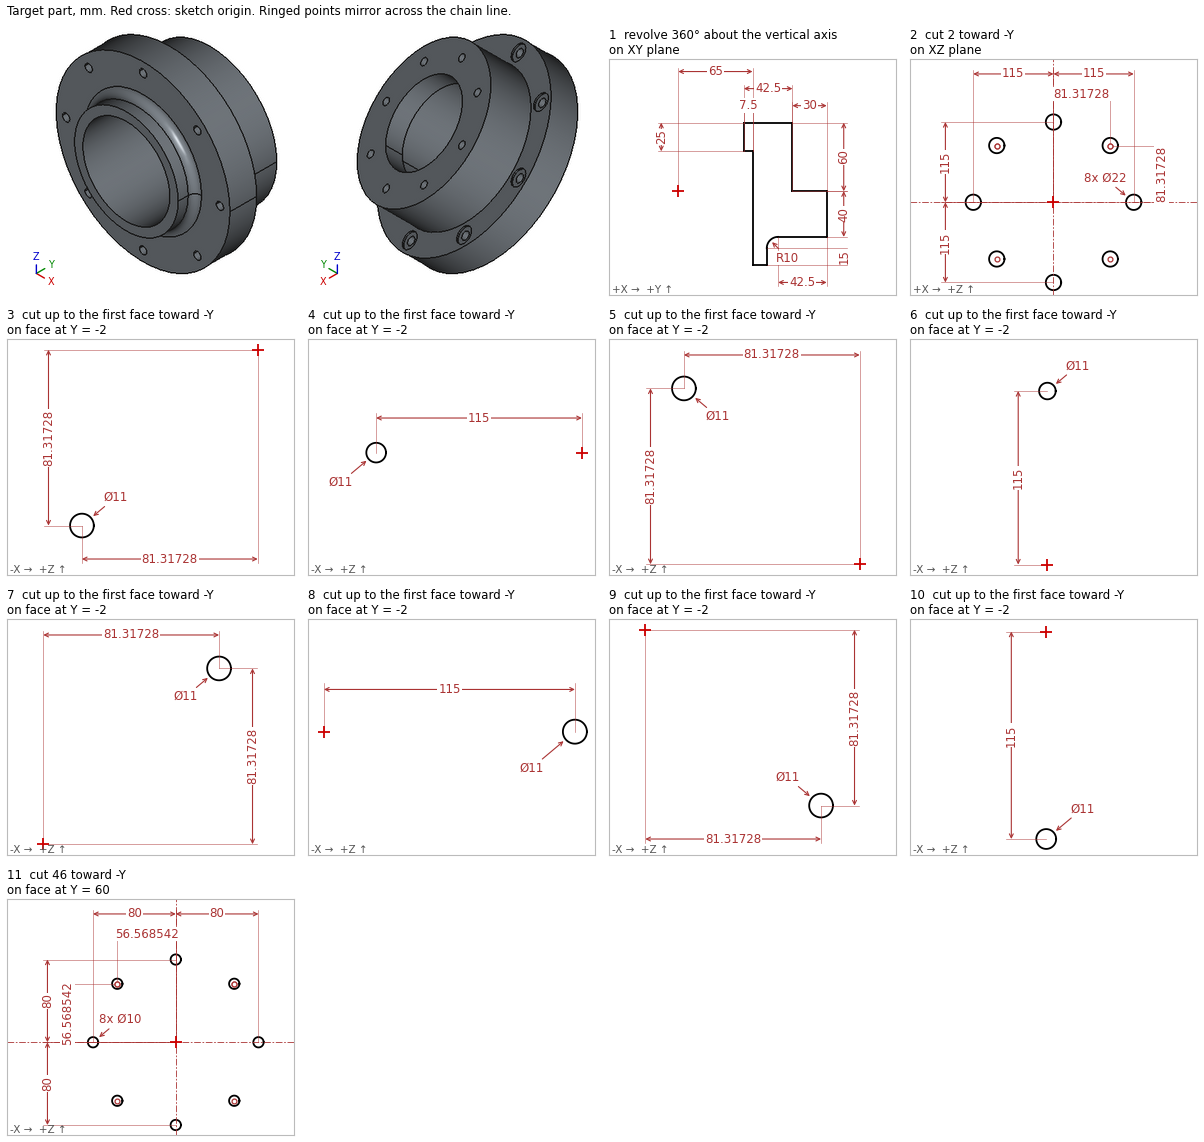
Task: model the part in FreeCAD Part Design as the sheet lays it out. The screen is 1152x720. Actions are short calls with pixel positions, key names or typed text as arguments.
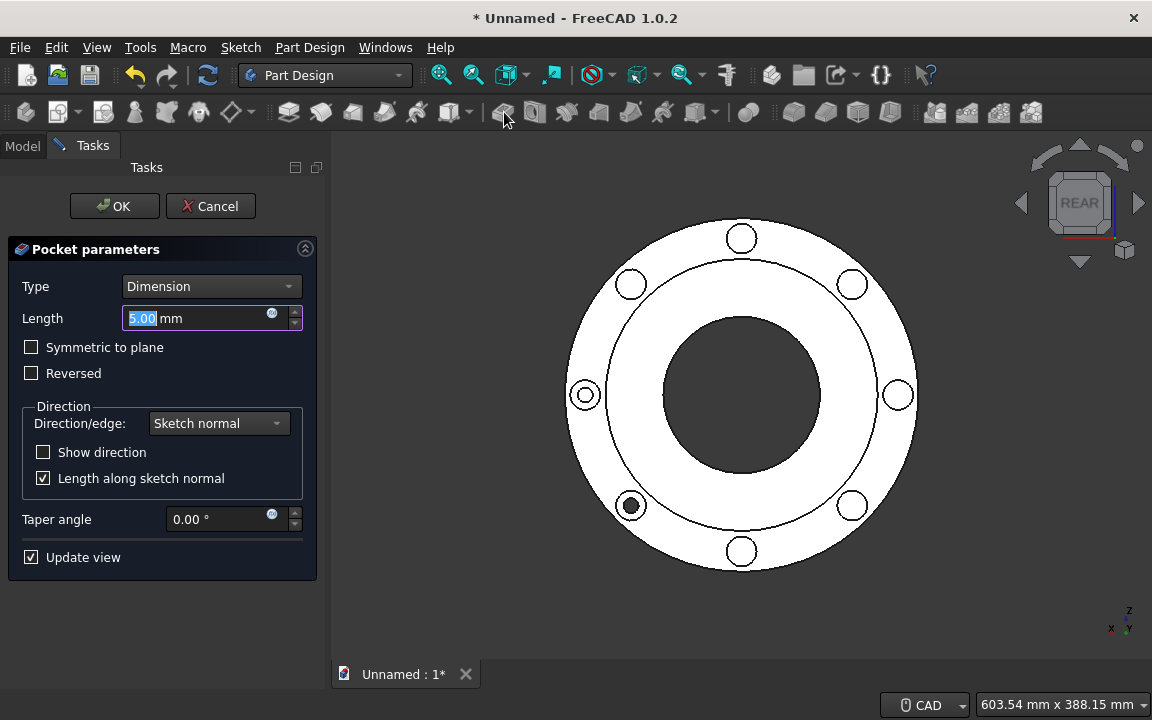
click(212, 286)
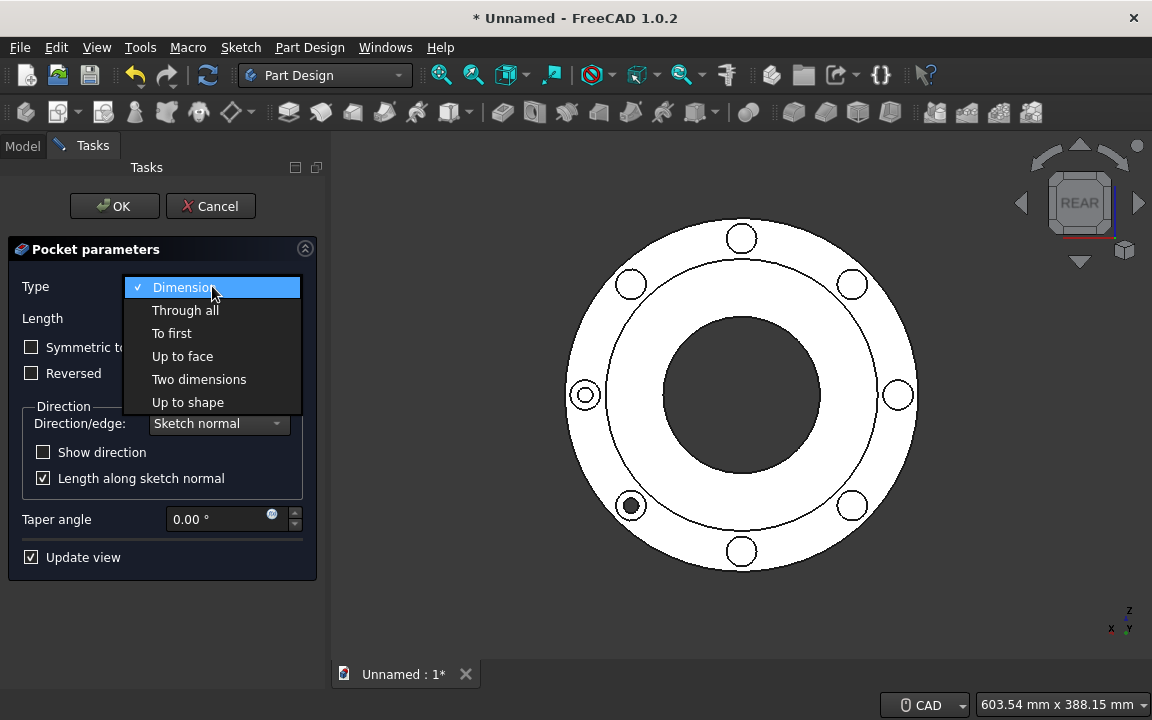
click(212, 334)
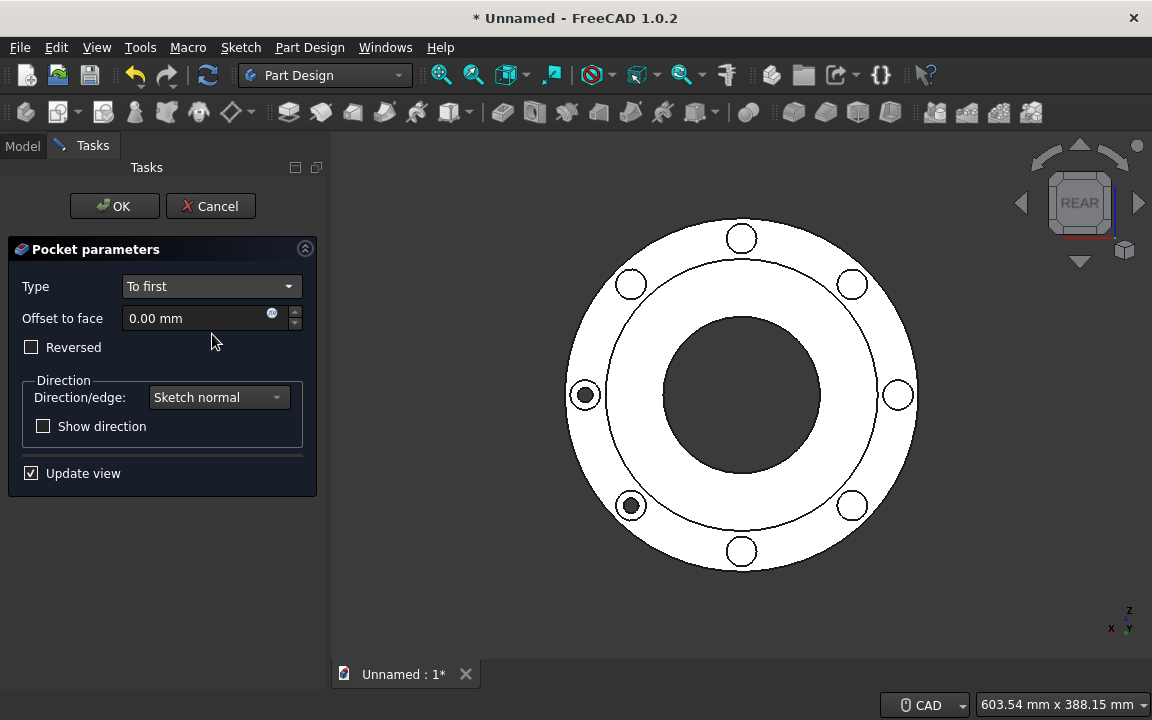
click(115, 206)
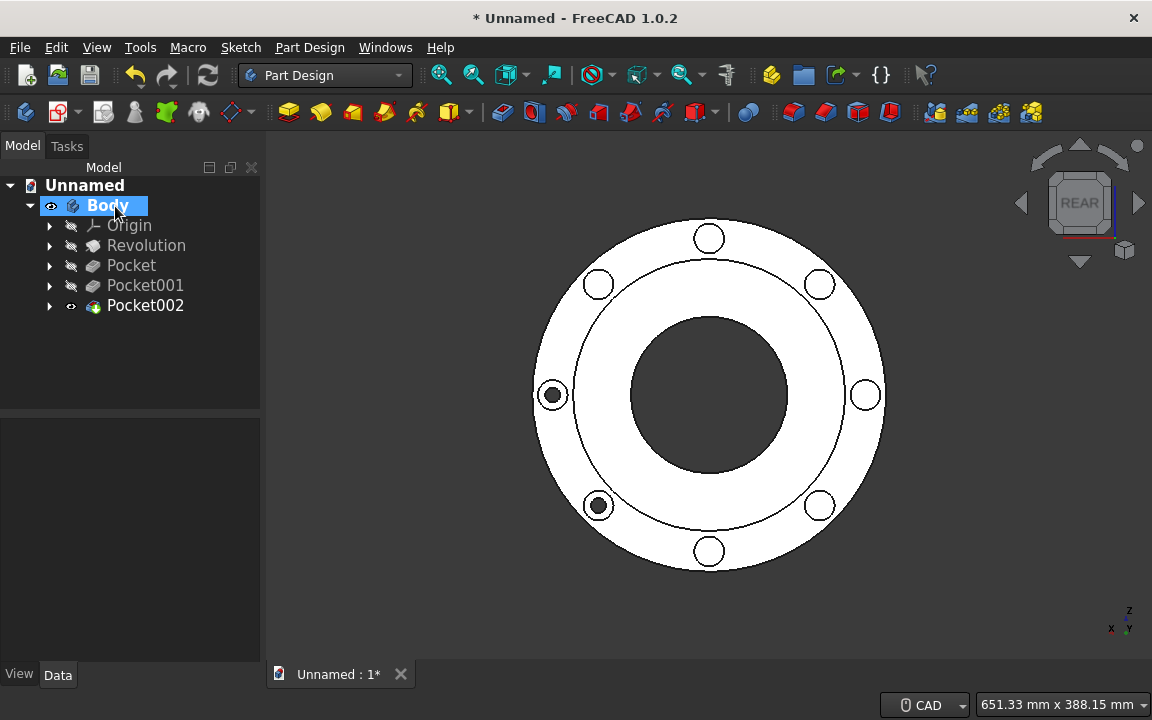
click(599, 283)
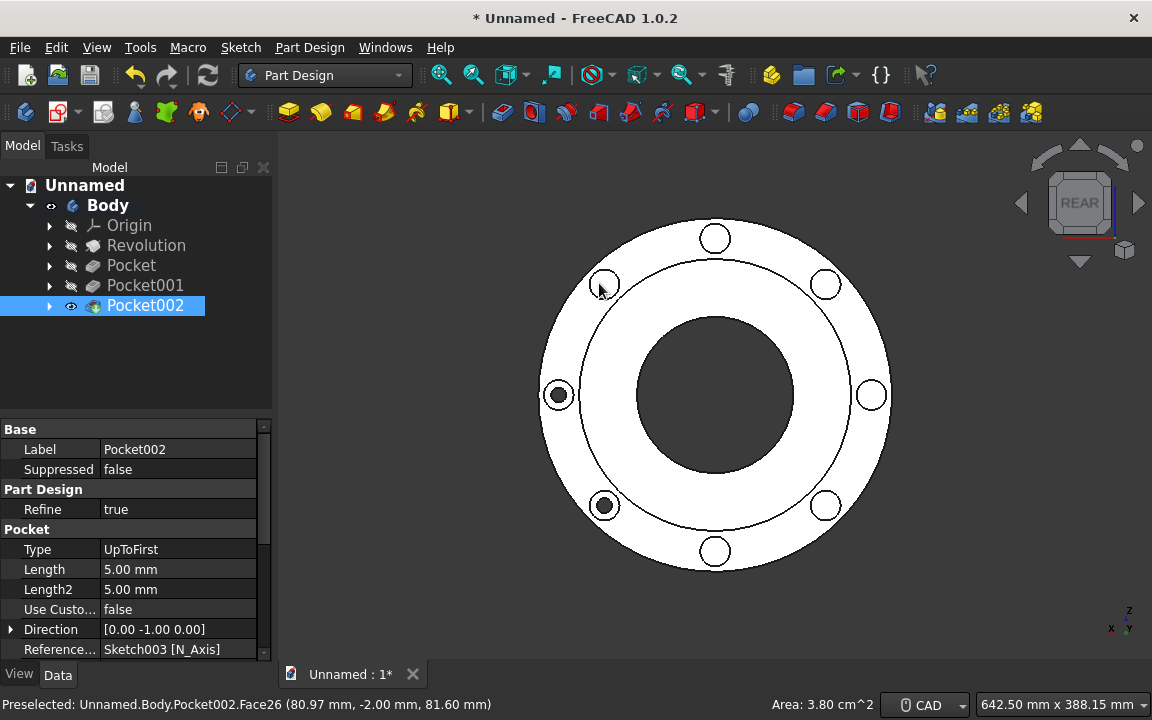
click(58, 112)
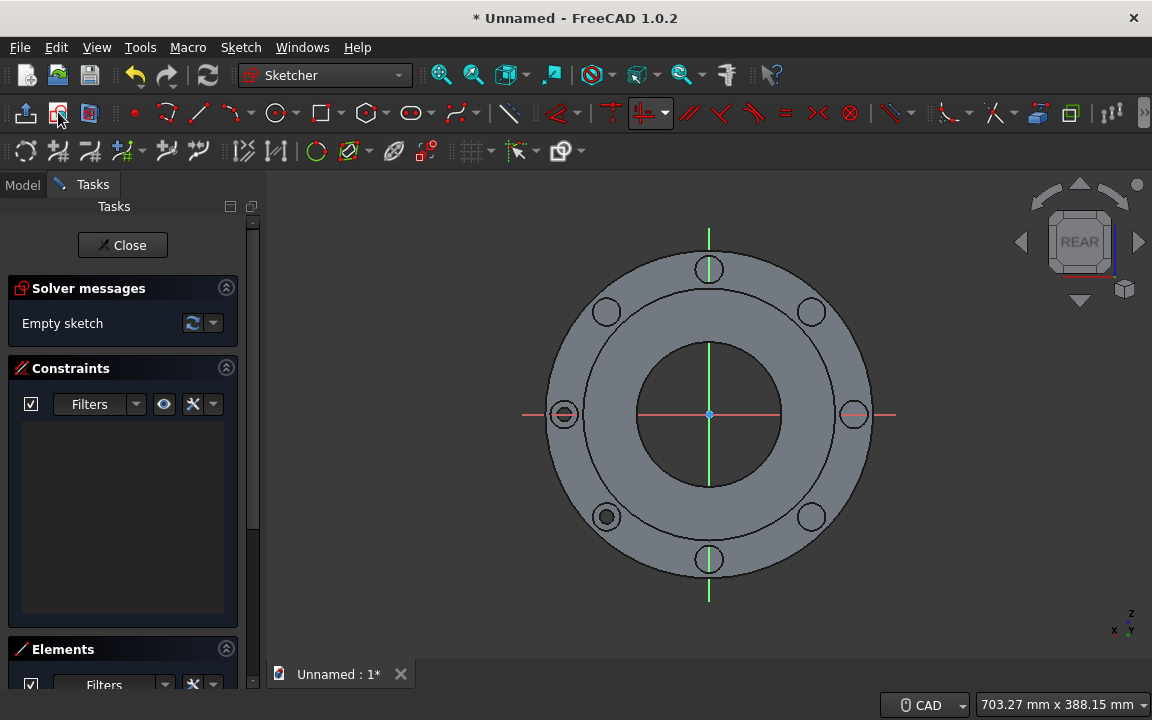
scroll(605, 307, up, 15)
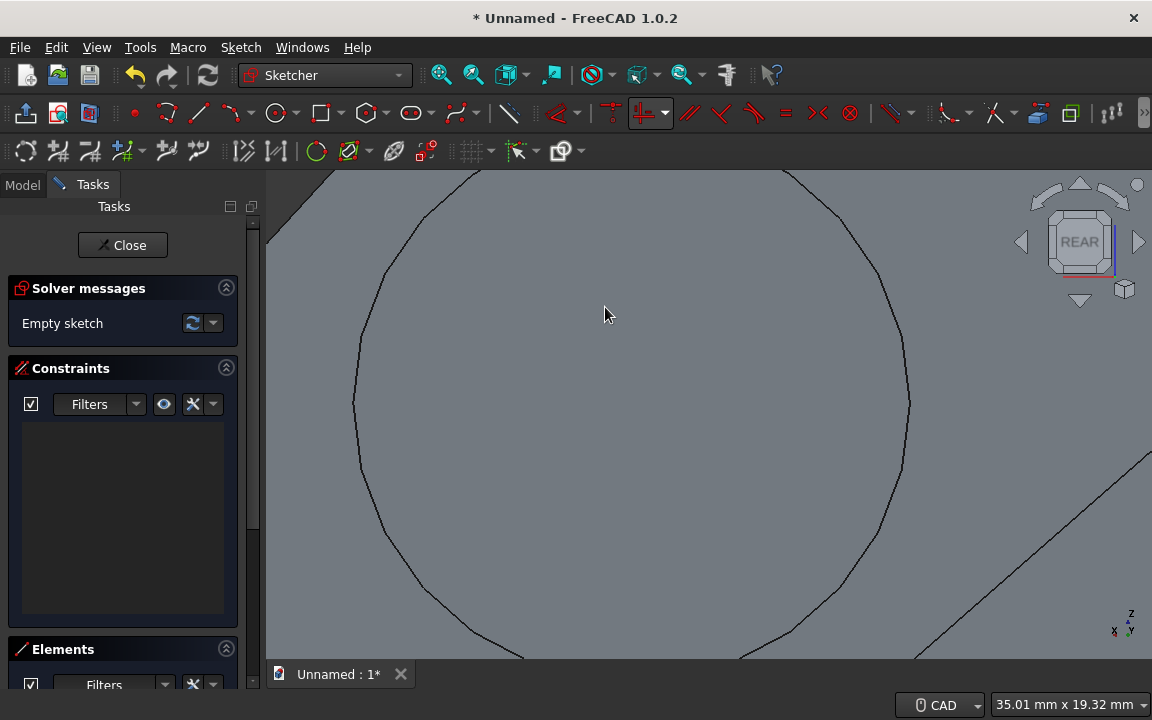
click(276, 114)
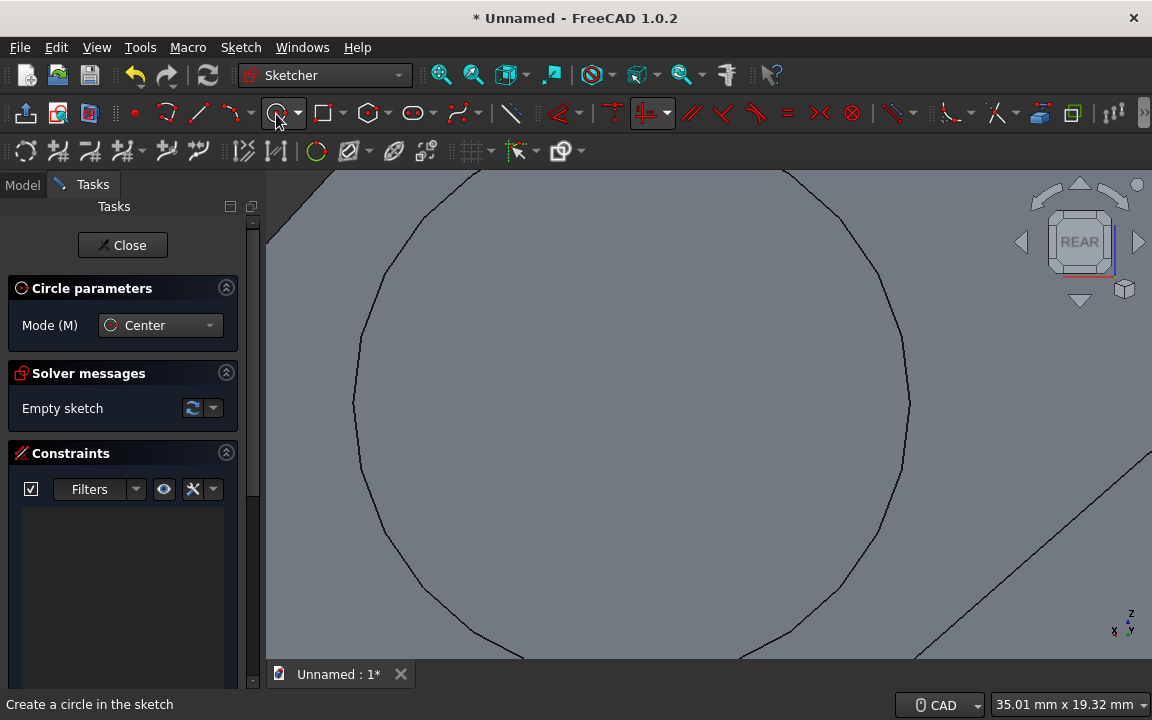
click(632, 403)
move(730, 305)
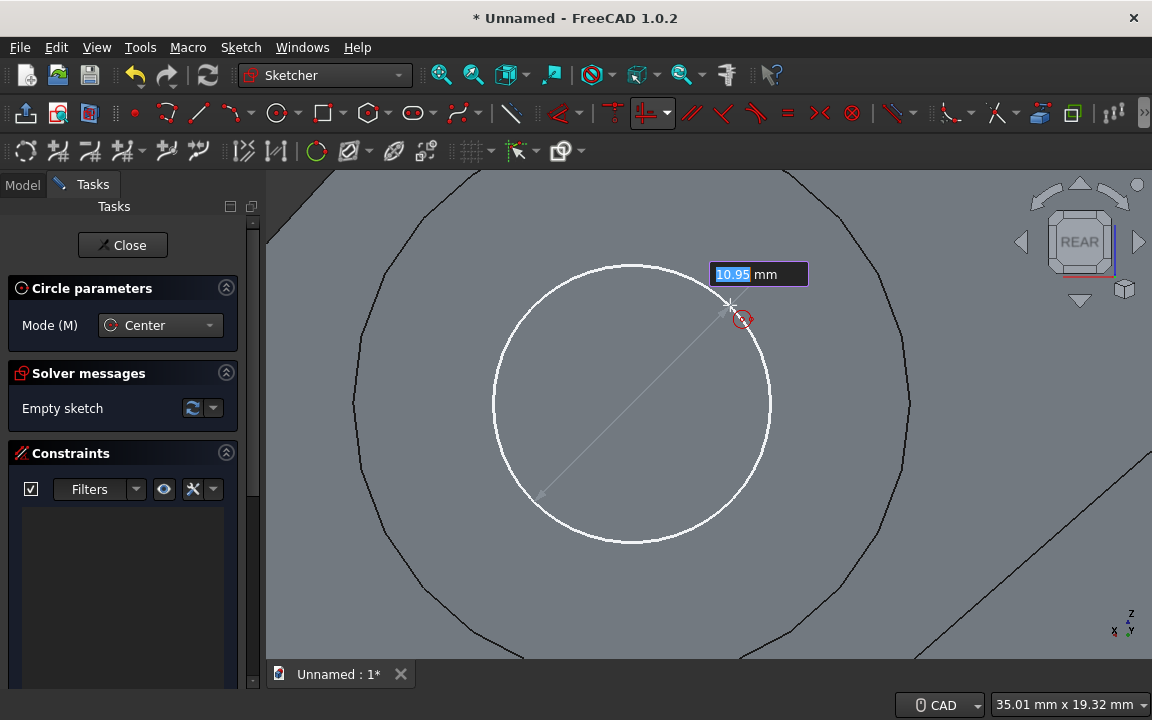
text(11)
key(Return)
key(Escape)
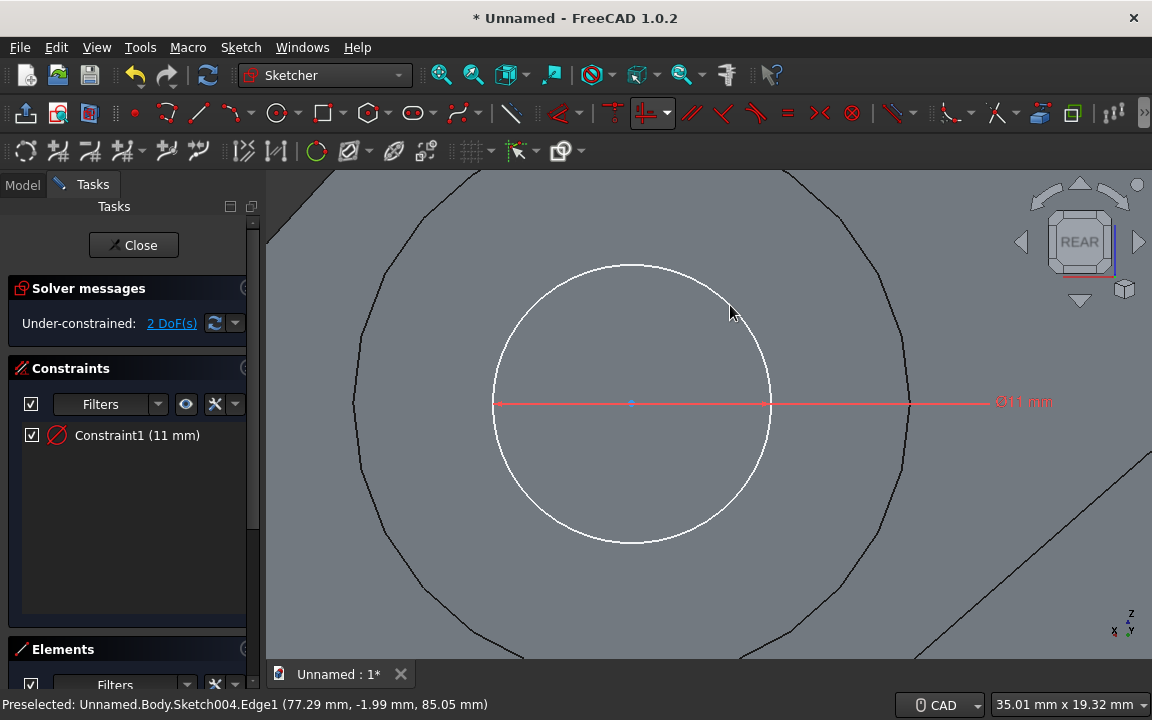
click(558, 114)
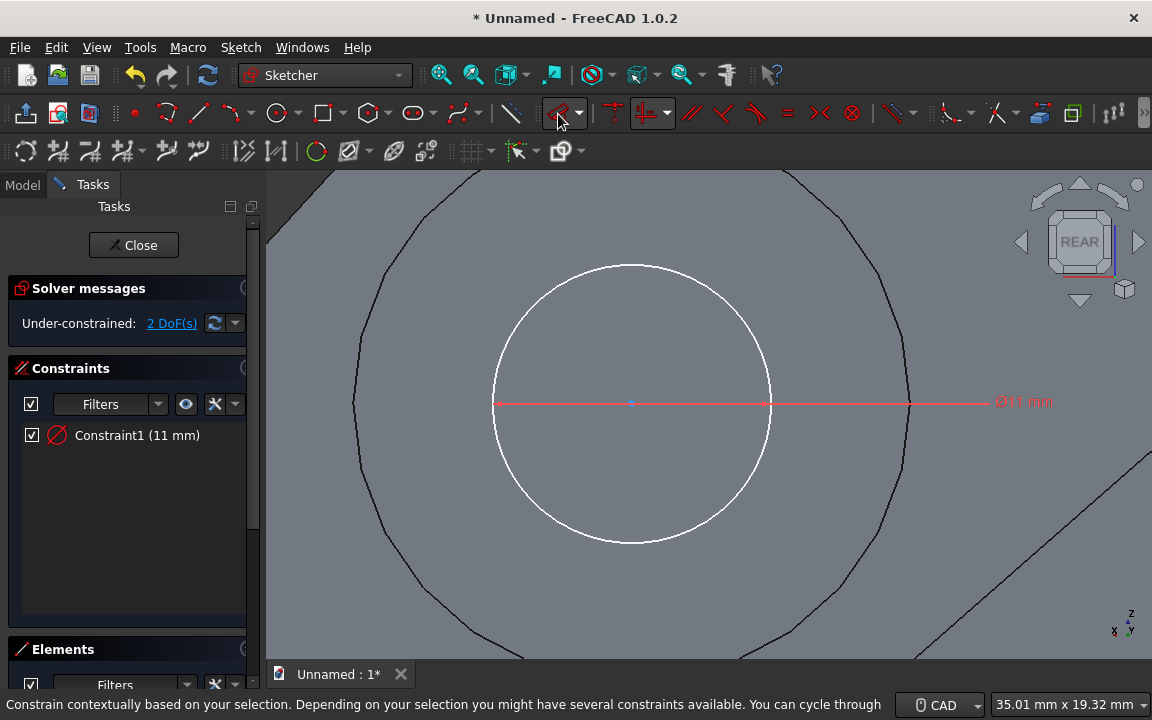
click(632, 404)
click(809, 370)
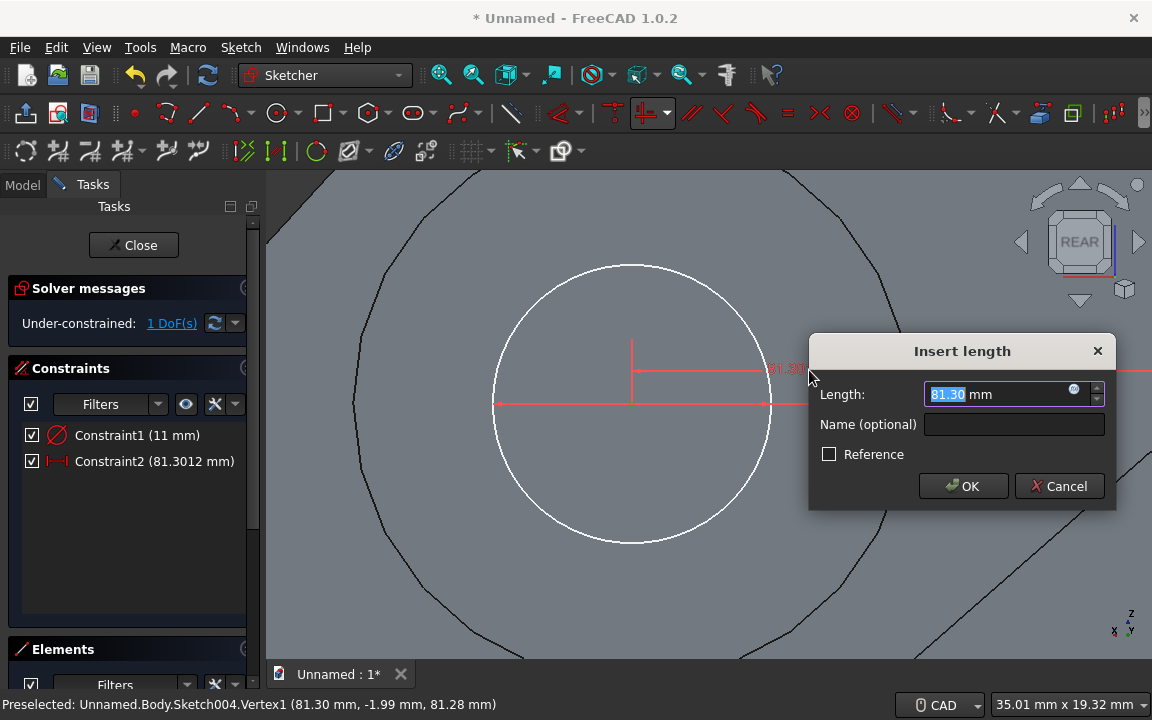
text(81.31728)
key(Return)